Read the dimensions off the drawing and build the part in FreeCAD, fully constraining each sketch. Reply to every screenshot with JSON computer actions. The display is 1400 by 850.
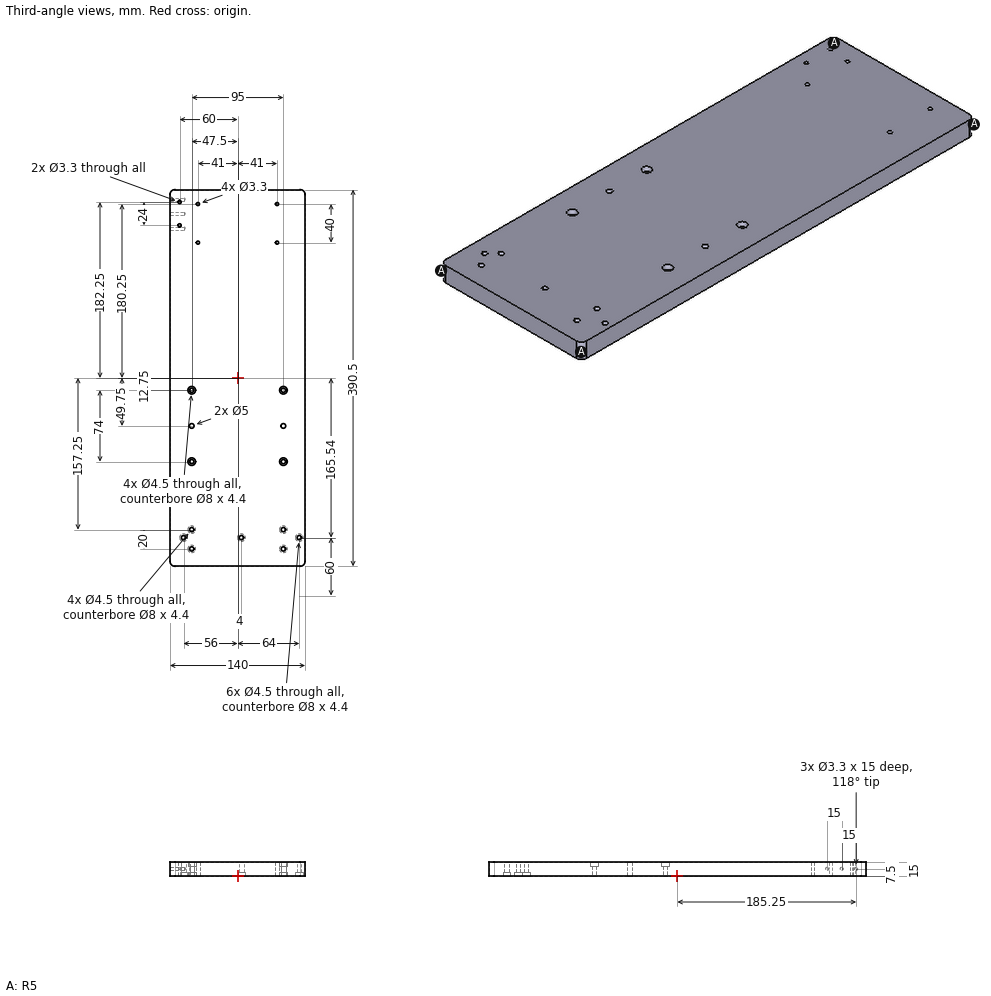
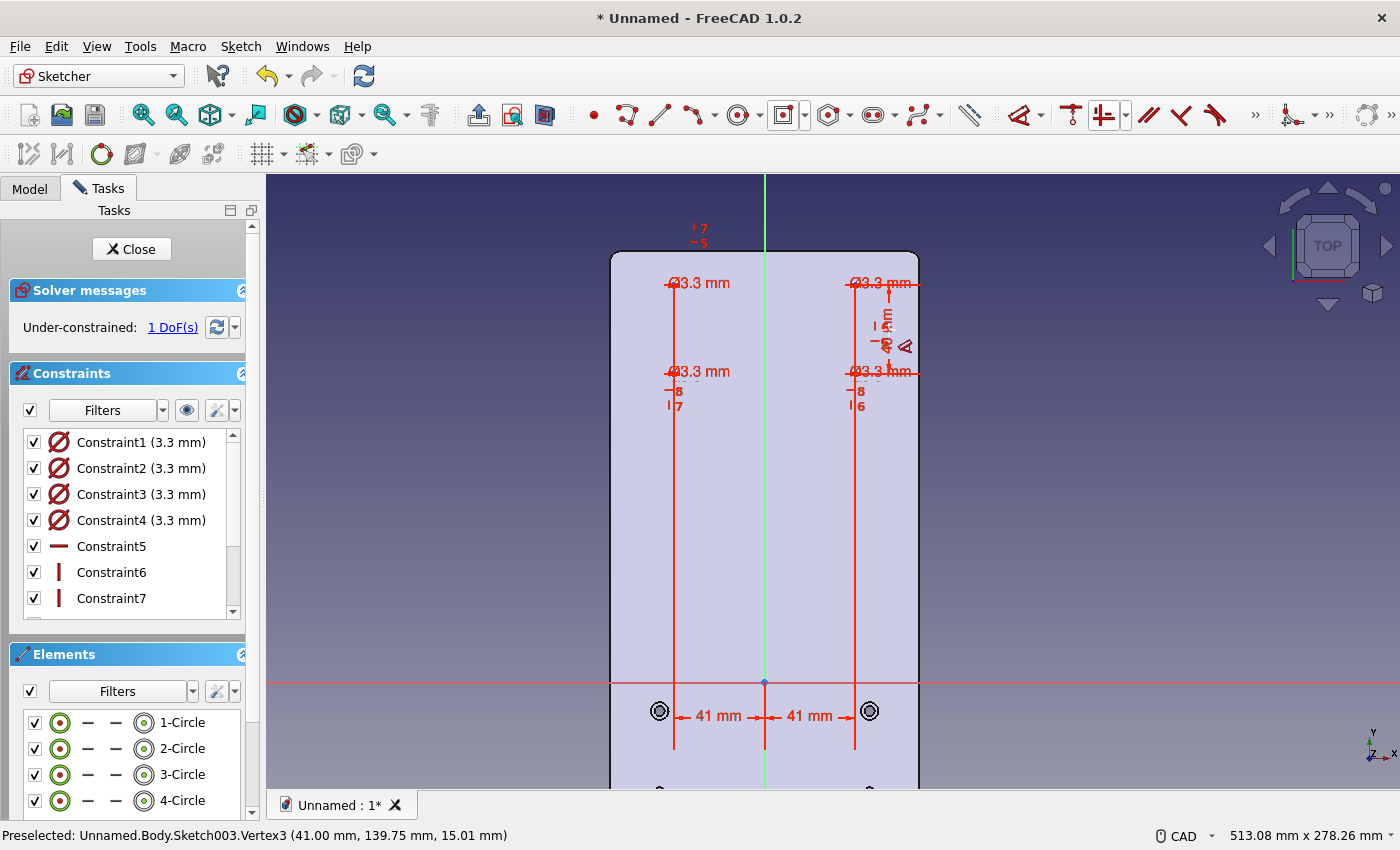
{"action": "left_click", "coordinate": [674, 285]}
{"action": "left_click", "coordinate": [640, 484]}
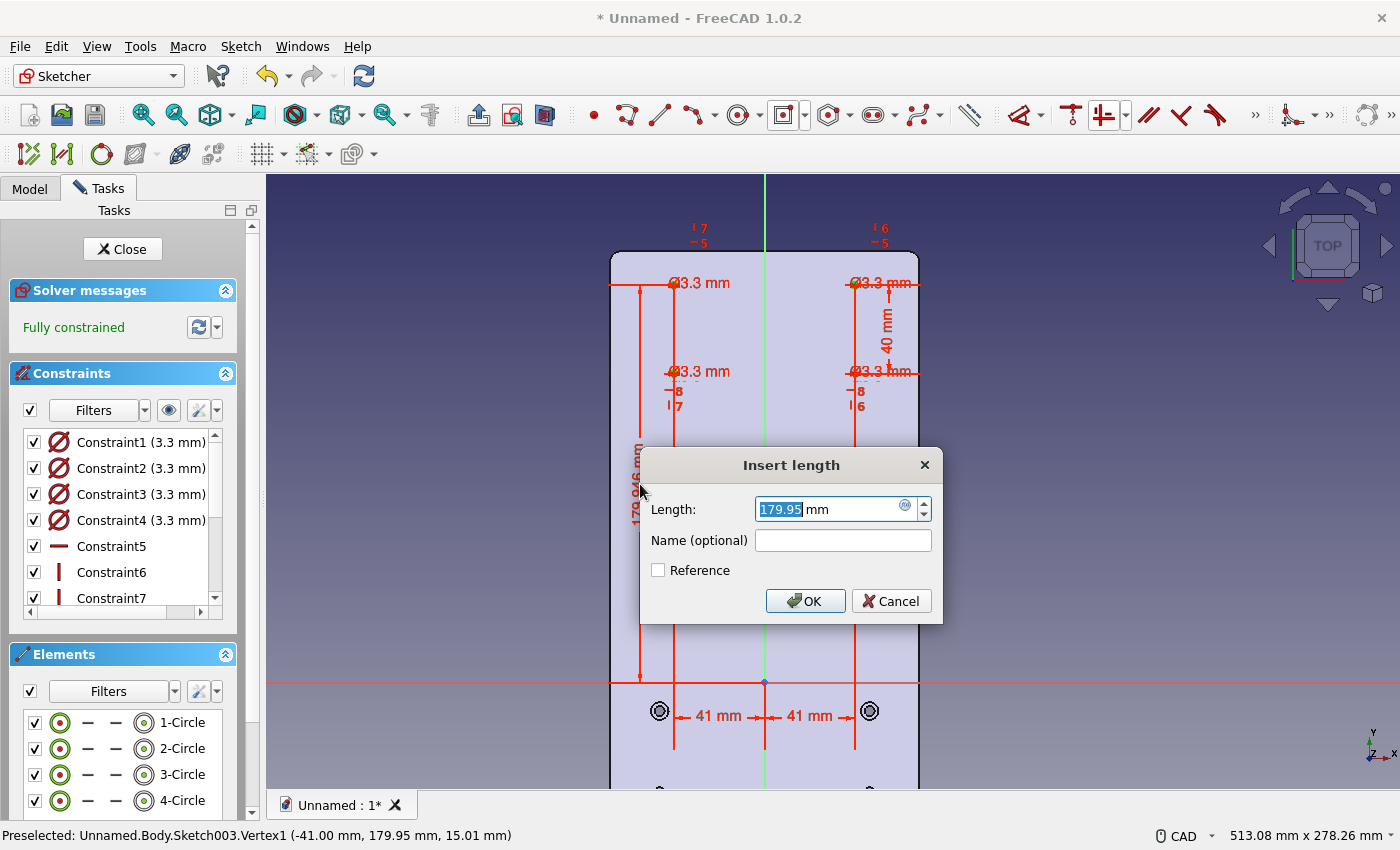
{"action": "type", "text": "180.25"}
{"action": "key", "text": "Return"}
{"action": "key", "text": "Escape"}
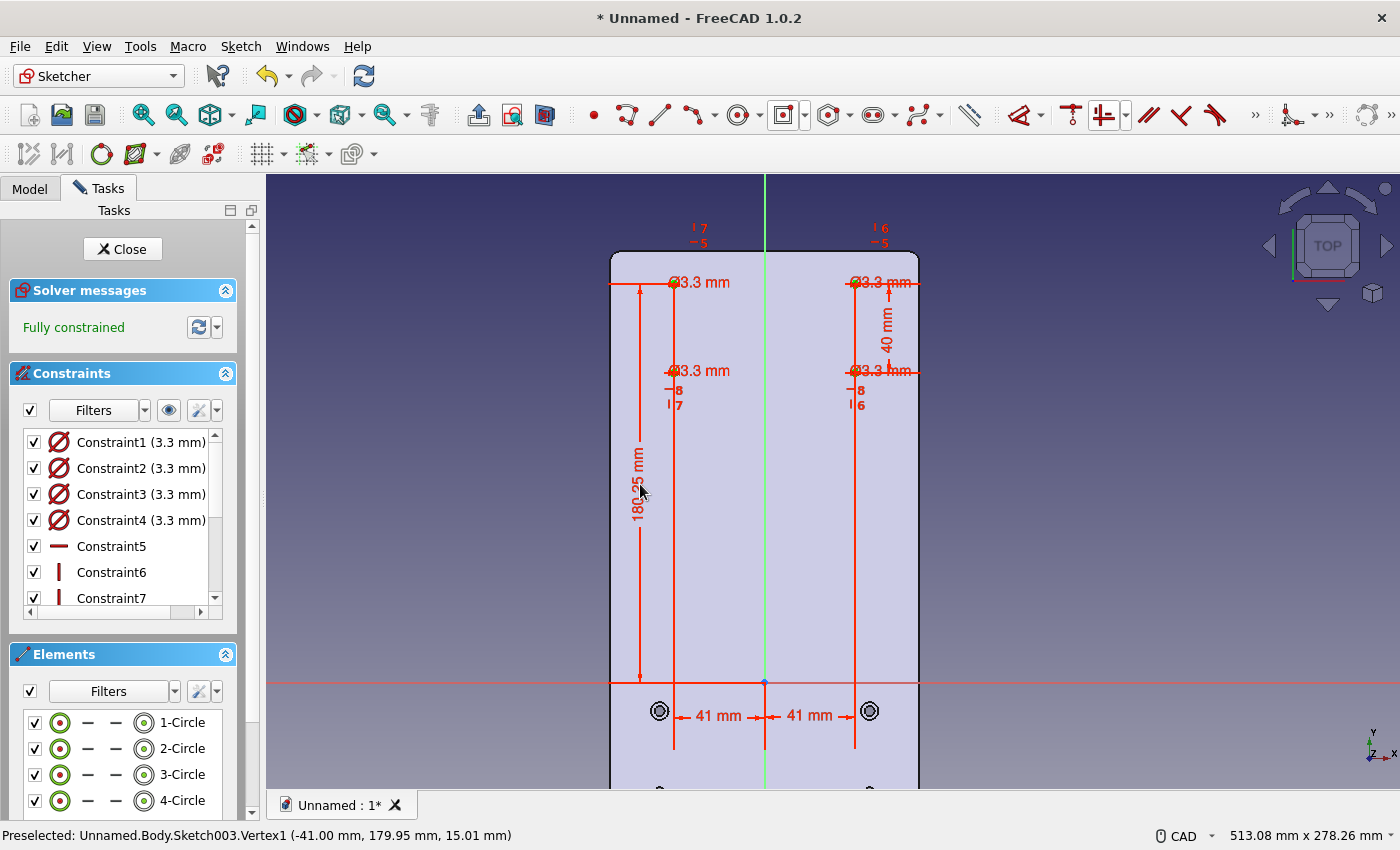
{"action": "left_click", "coordinate": [123, 249]}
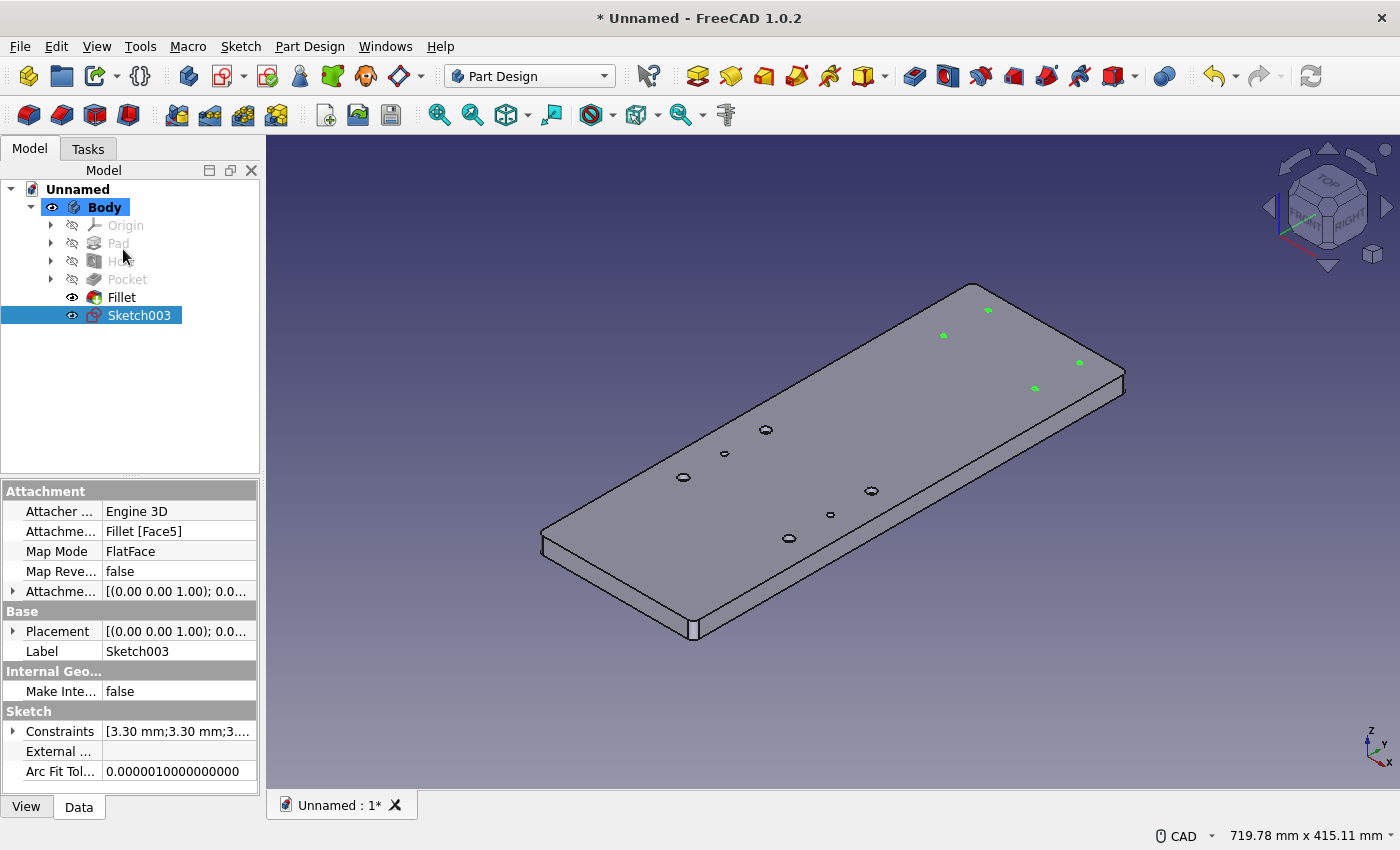
{"action": "left_click", "coordinate": [915, 76]}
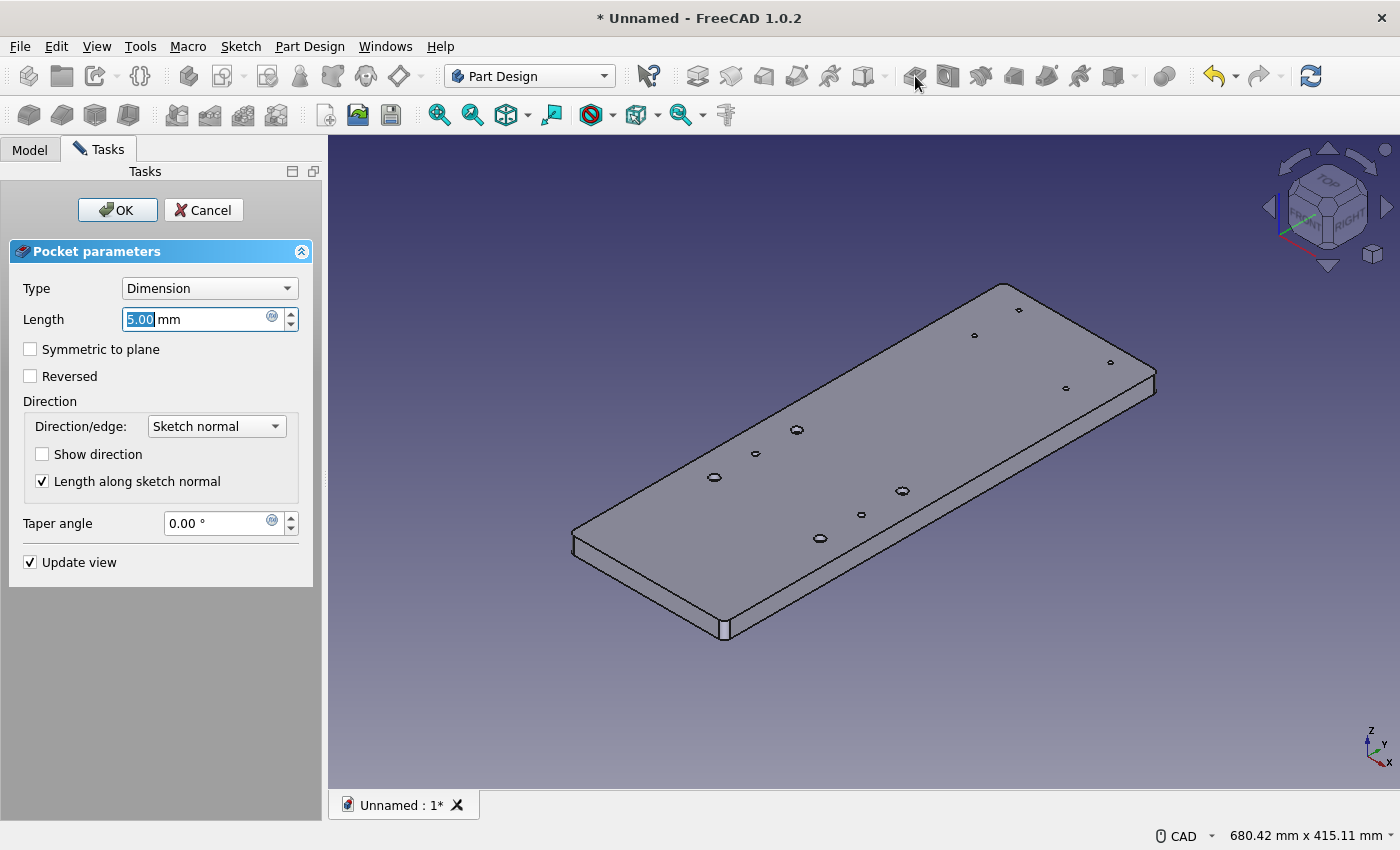
{"action": "left_click", "coordinate": [210, 288]}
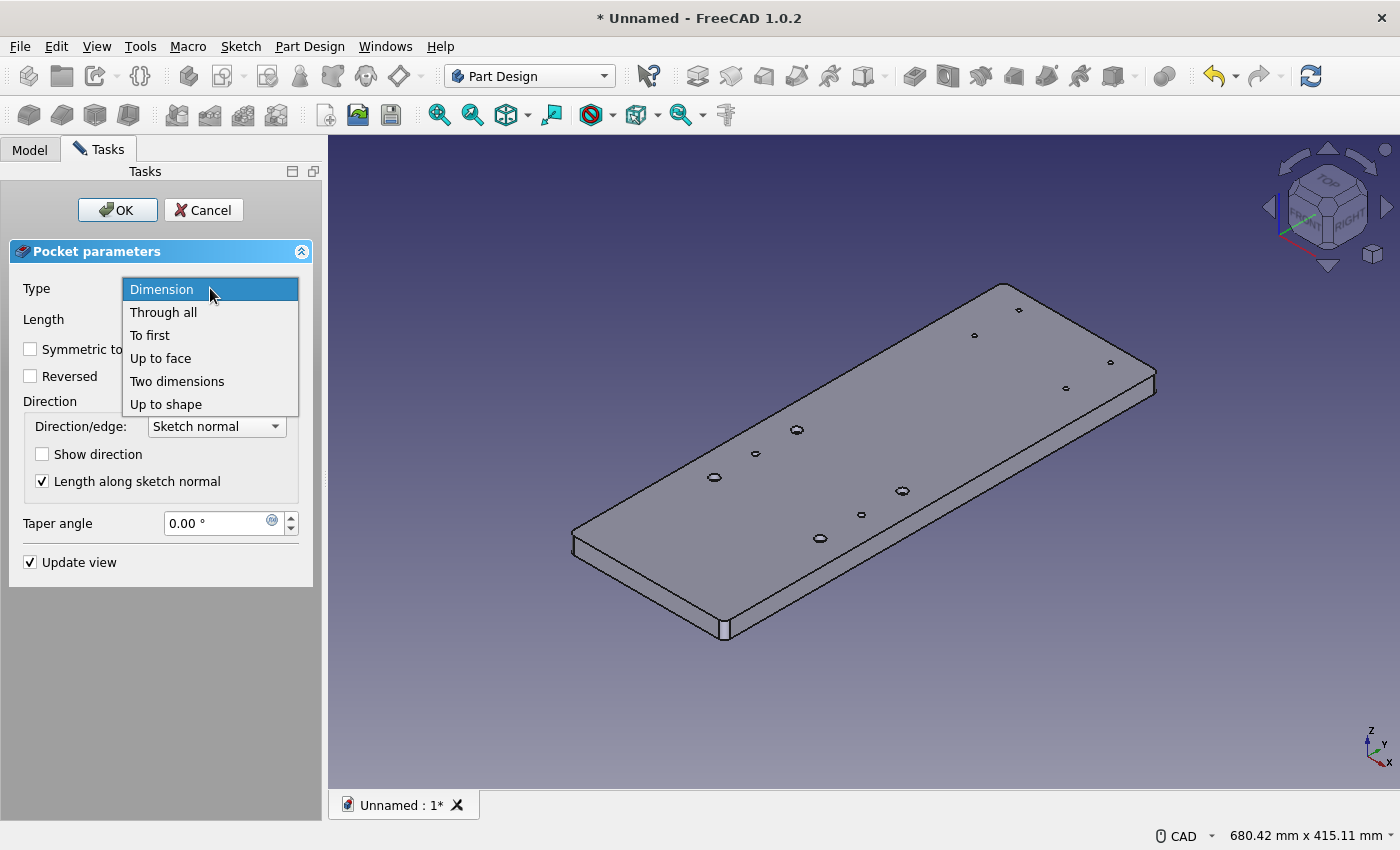
{"action": "left_click", "coordinate": [208, 312]}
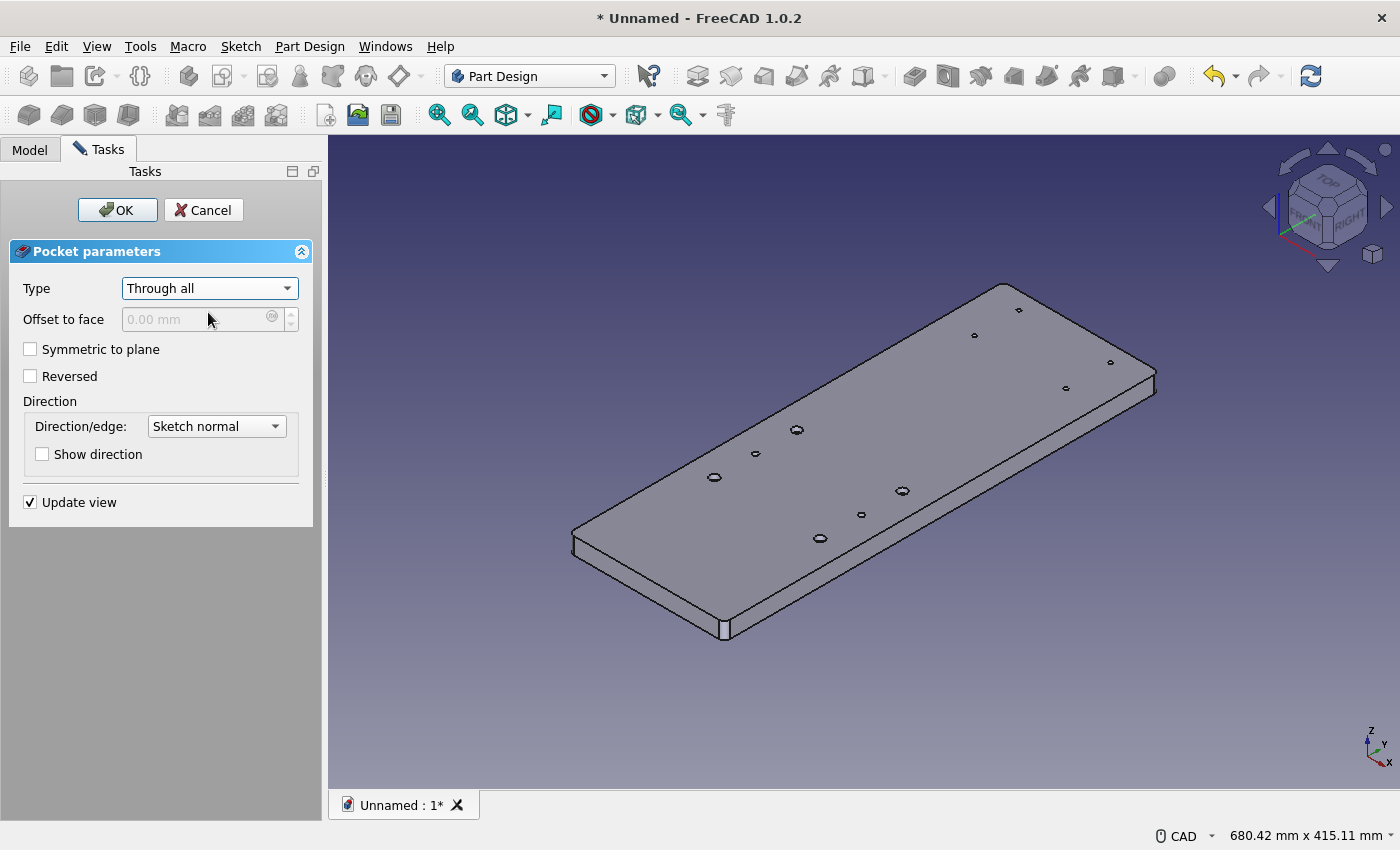
{"action": "left_click", "coordinate": [118, 210]}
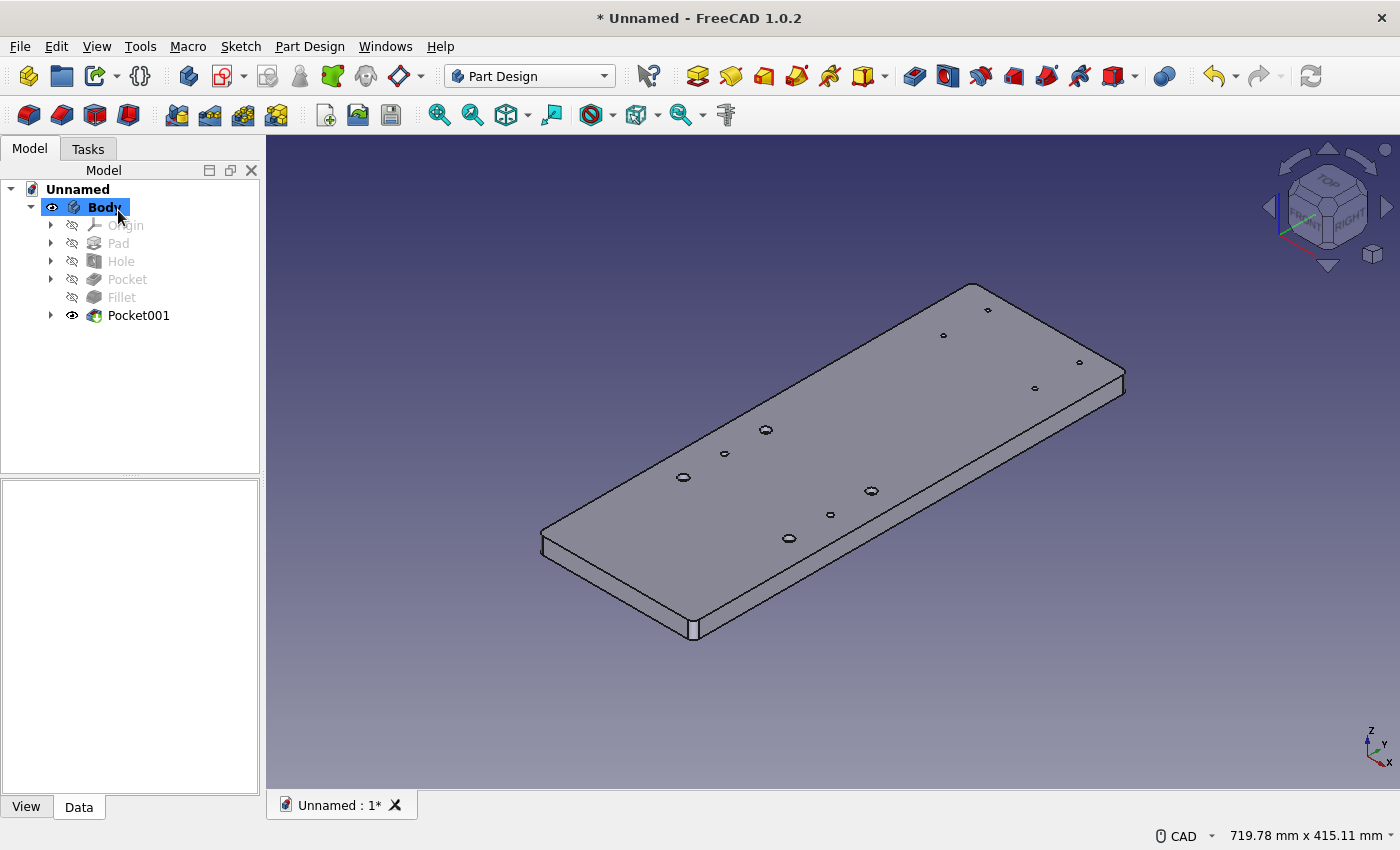
{"action": "left_click", "coordinate": [222, 76]}